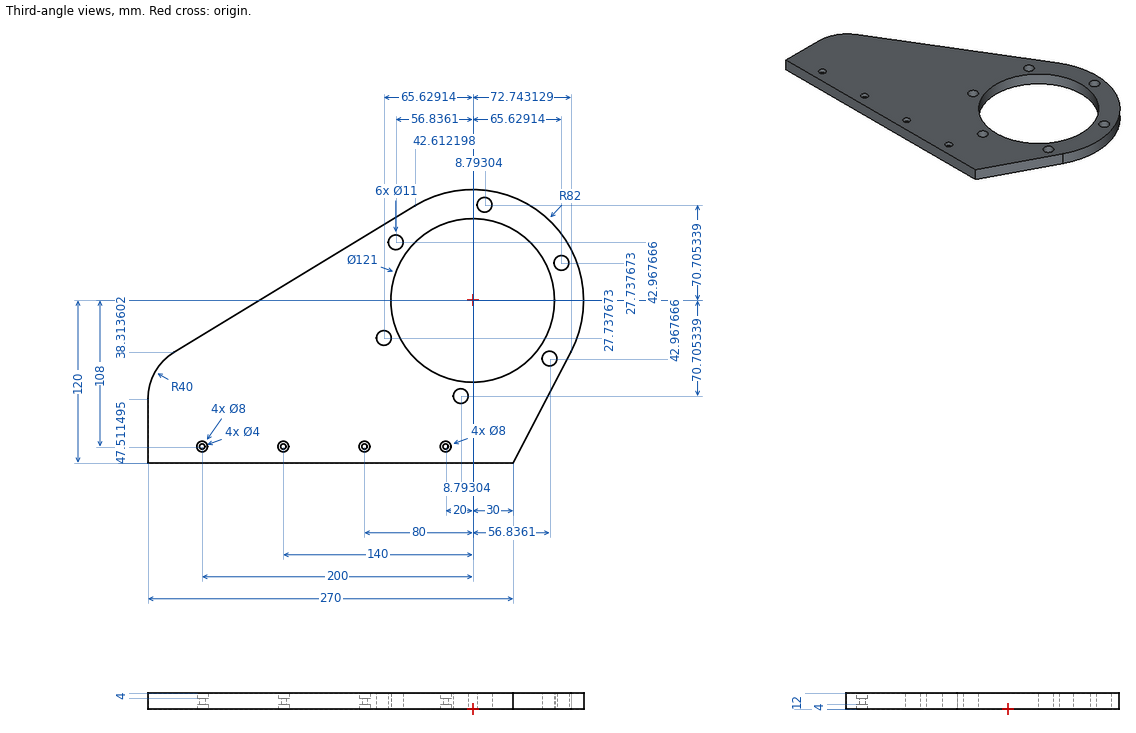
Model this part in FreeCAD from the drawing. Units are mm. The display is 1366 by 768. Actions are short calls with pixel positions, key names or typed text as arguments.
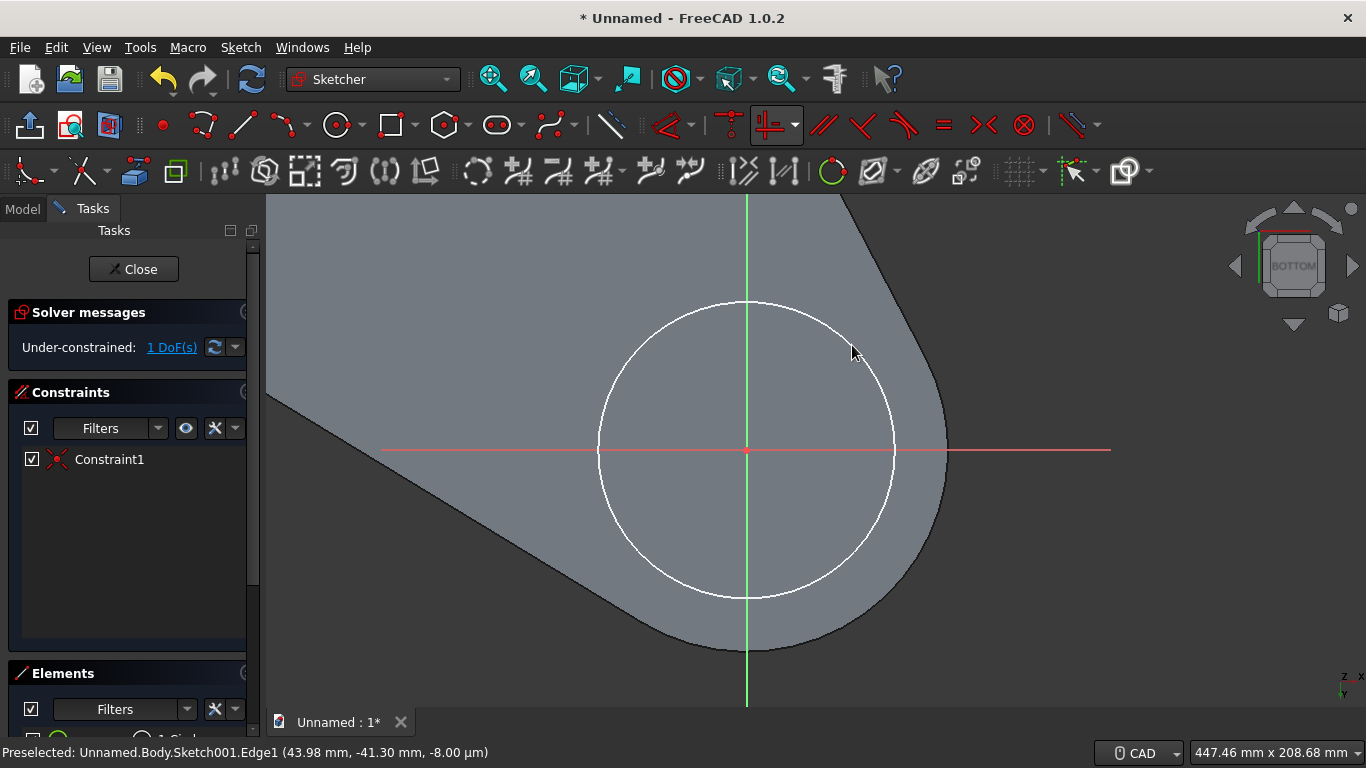
click(666, 126)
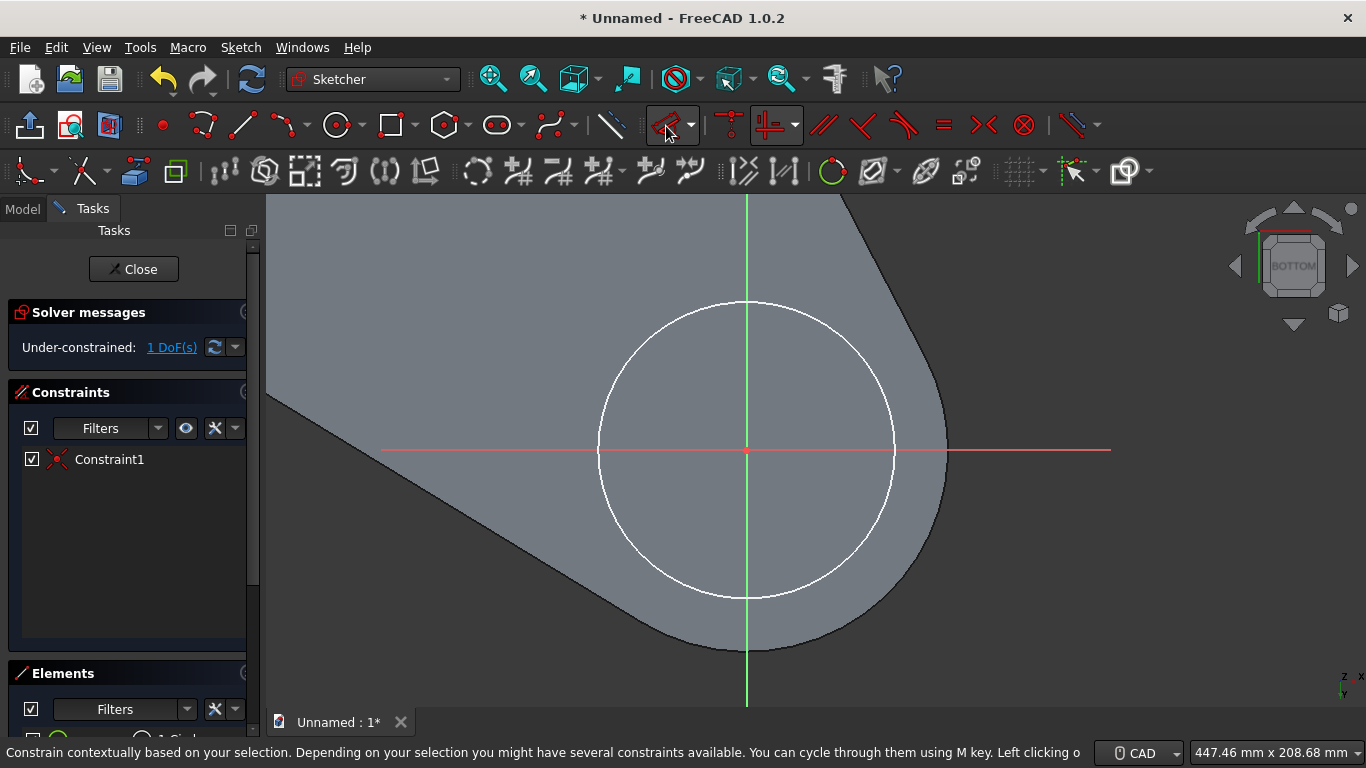
click(851, 345)
click(874, 322)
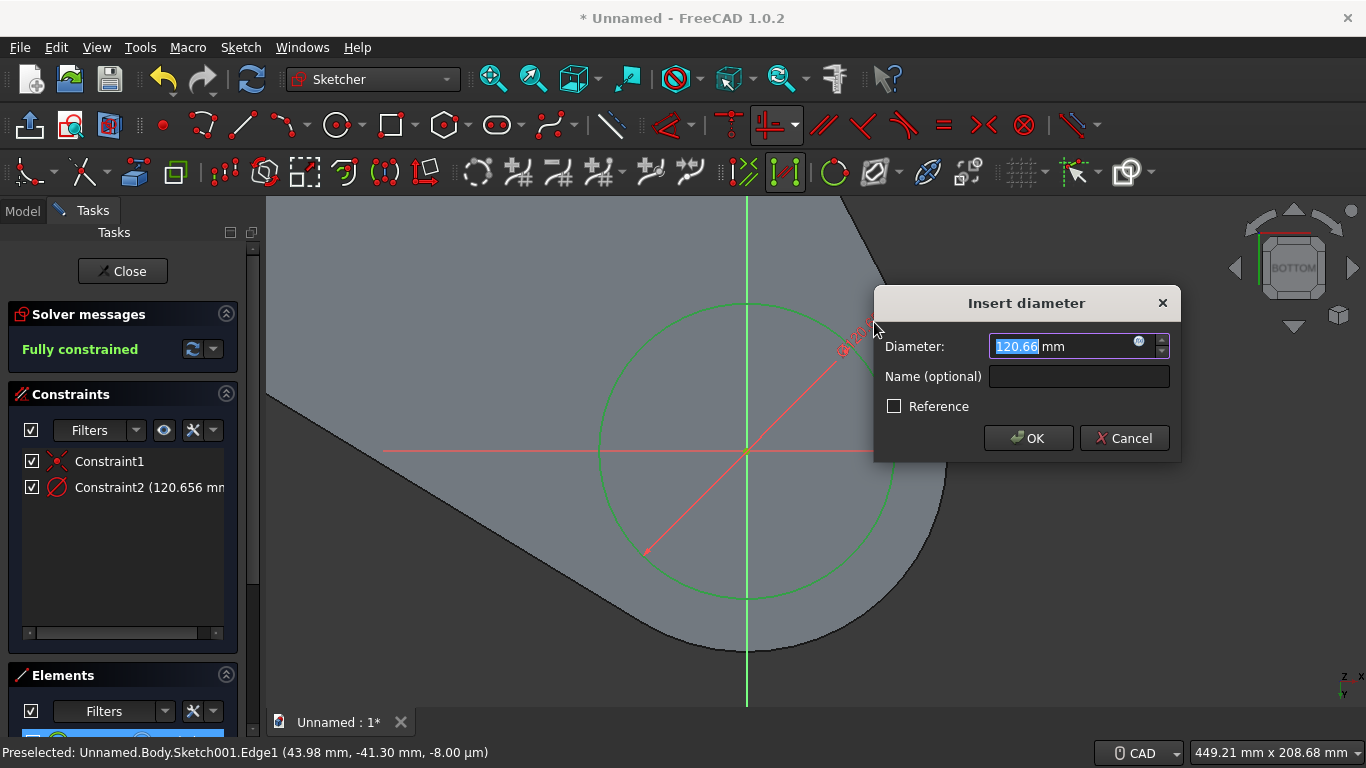
text(121)
key(Return)
key(Escape)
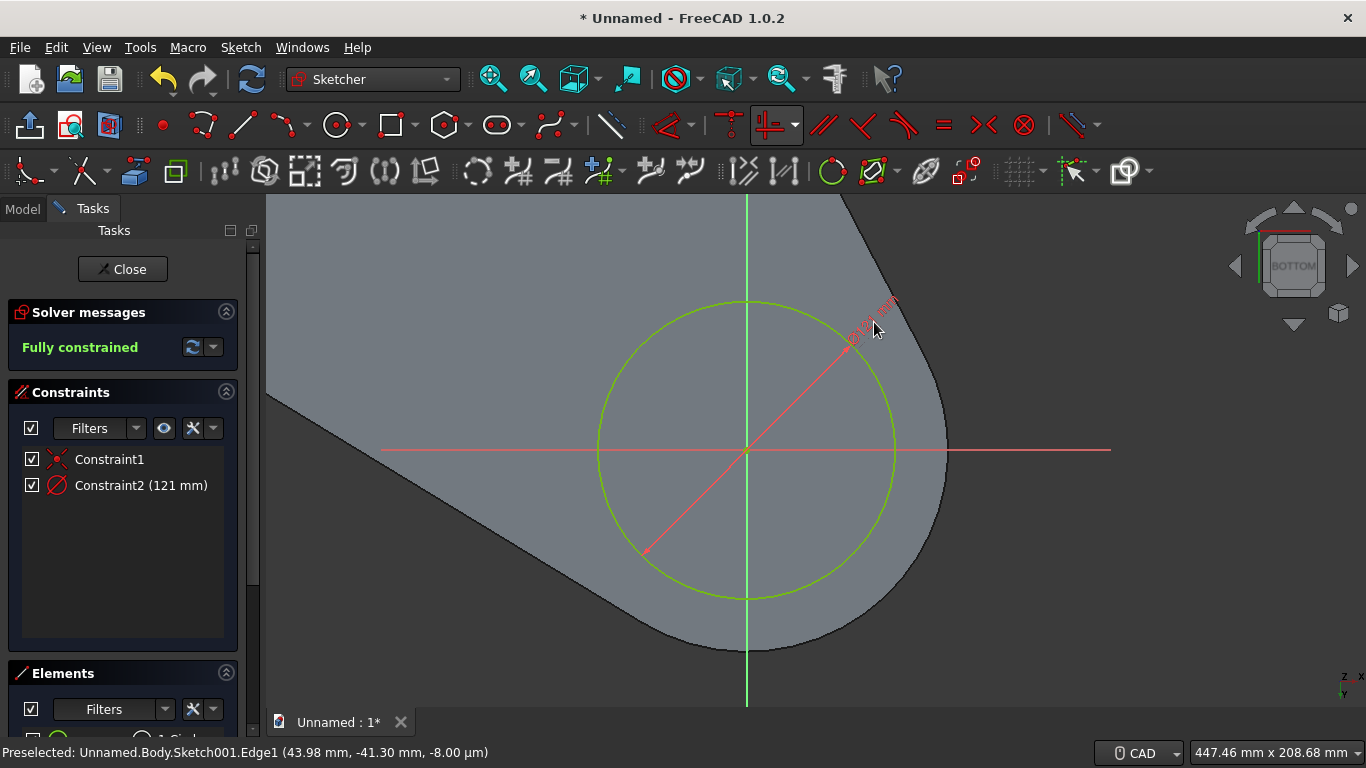
click(123, 269)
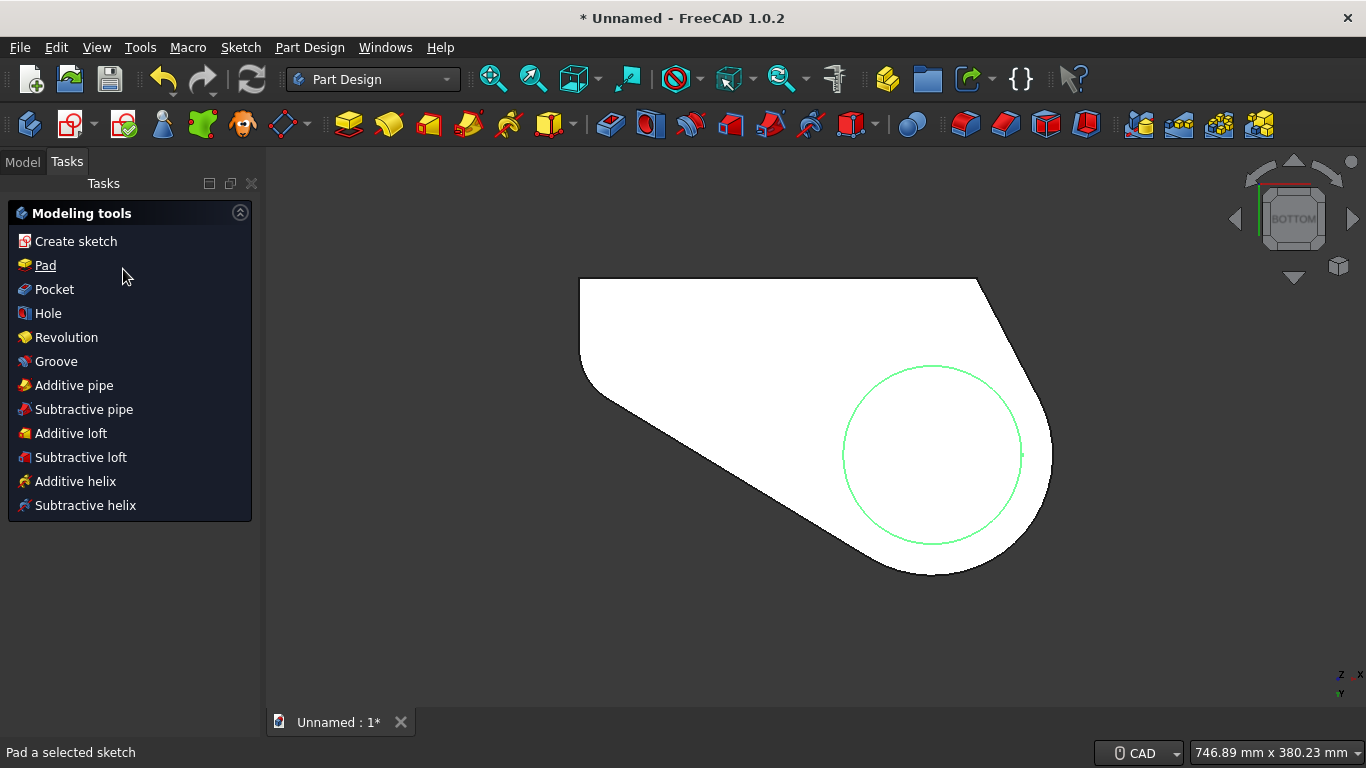
click(612, 124)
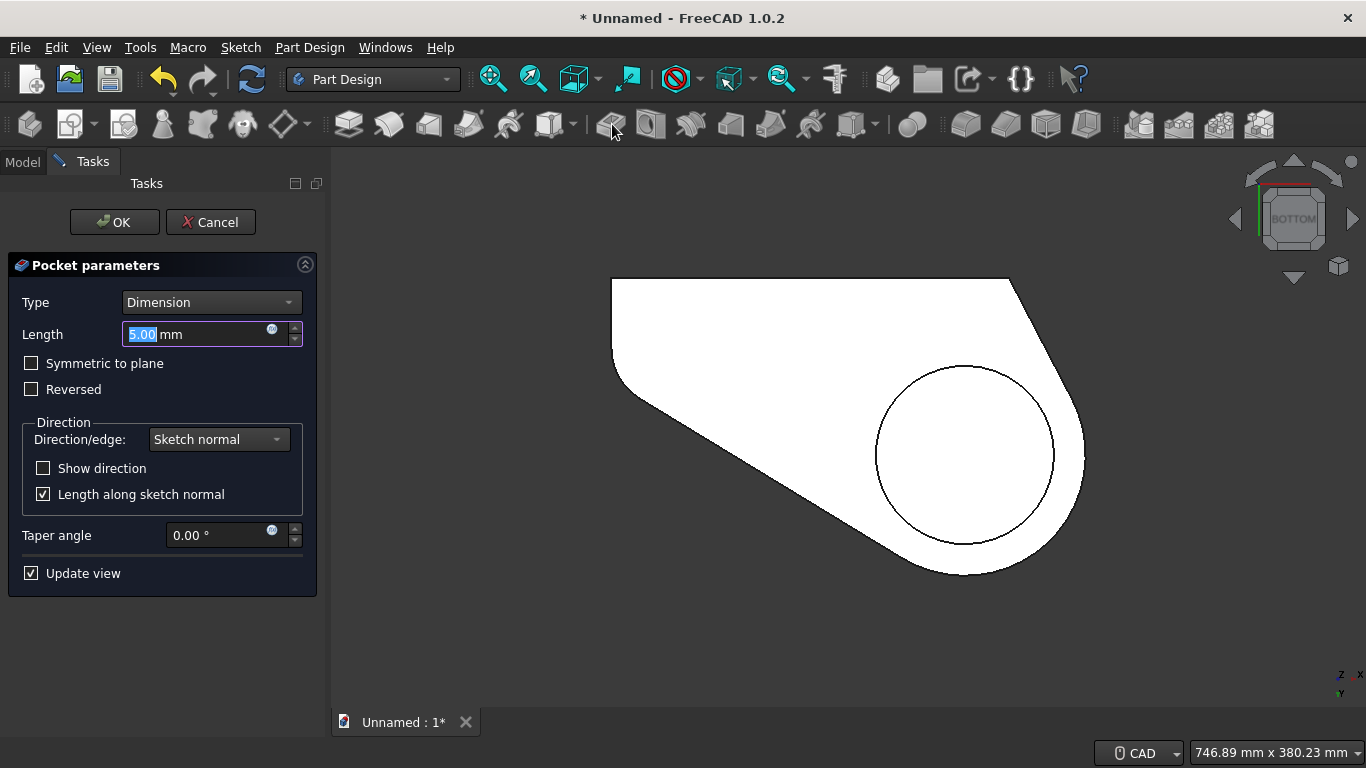
click(212, 302)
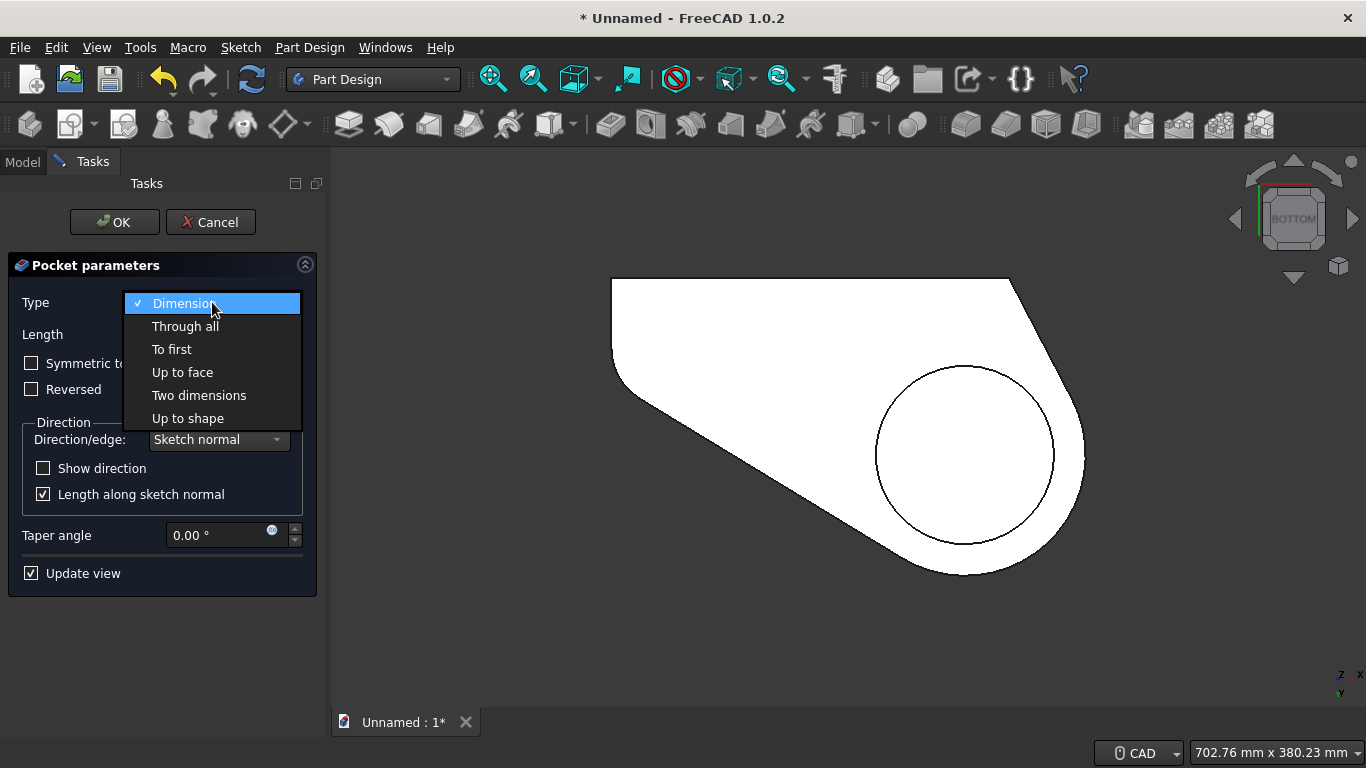
click(212, 326)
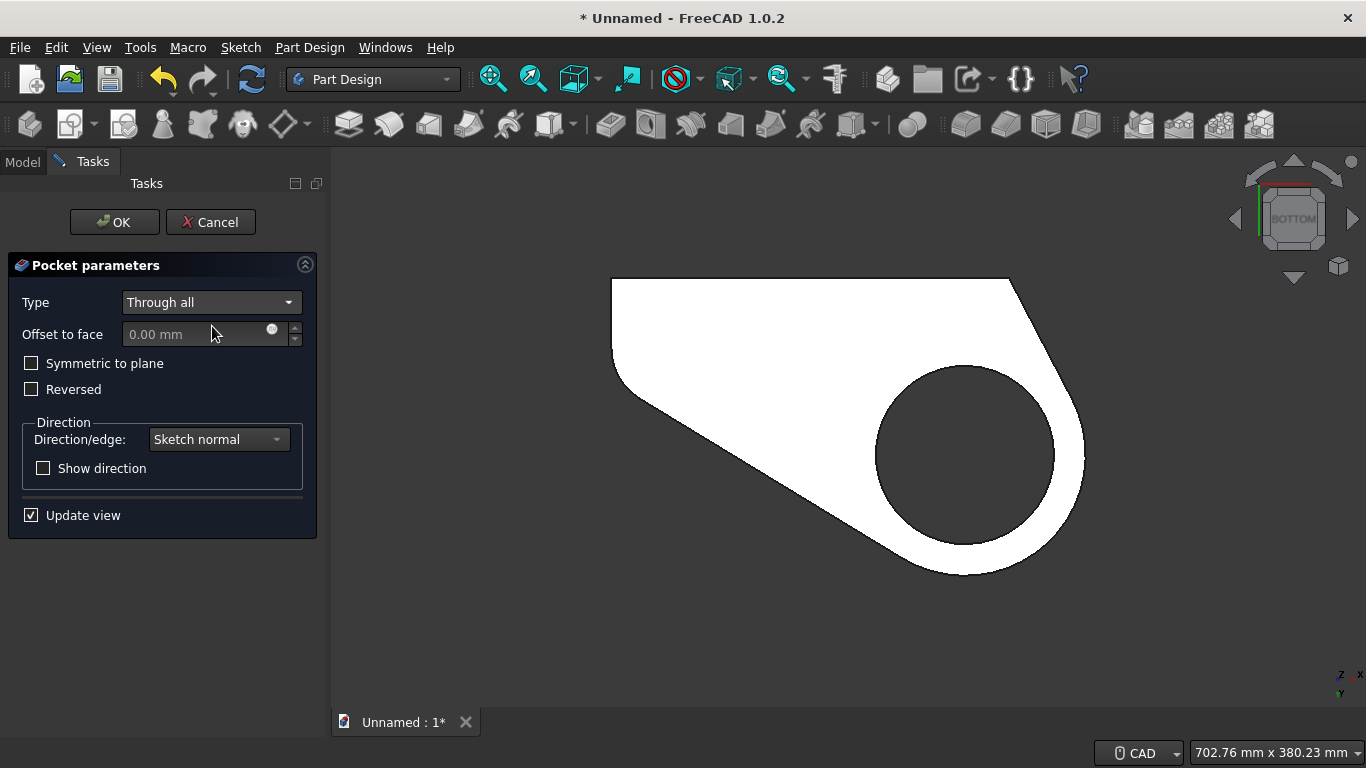
click(115, 222)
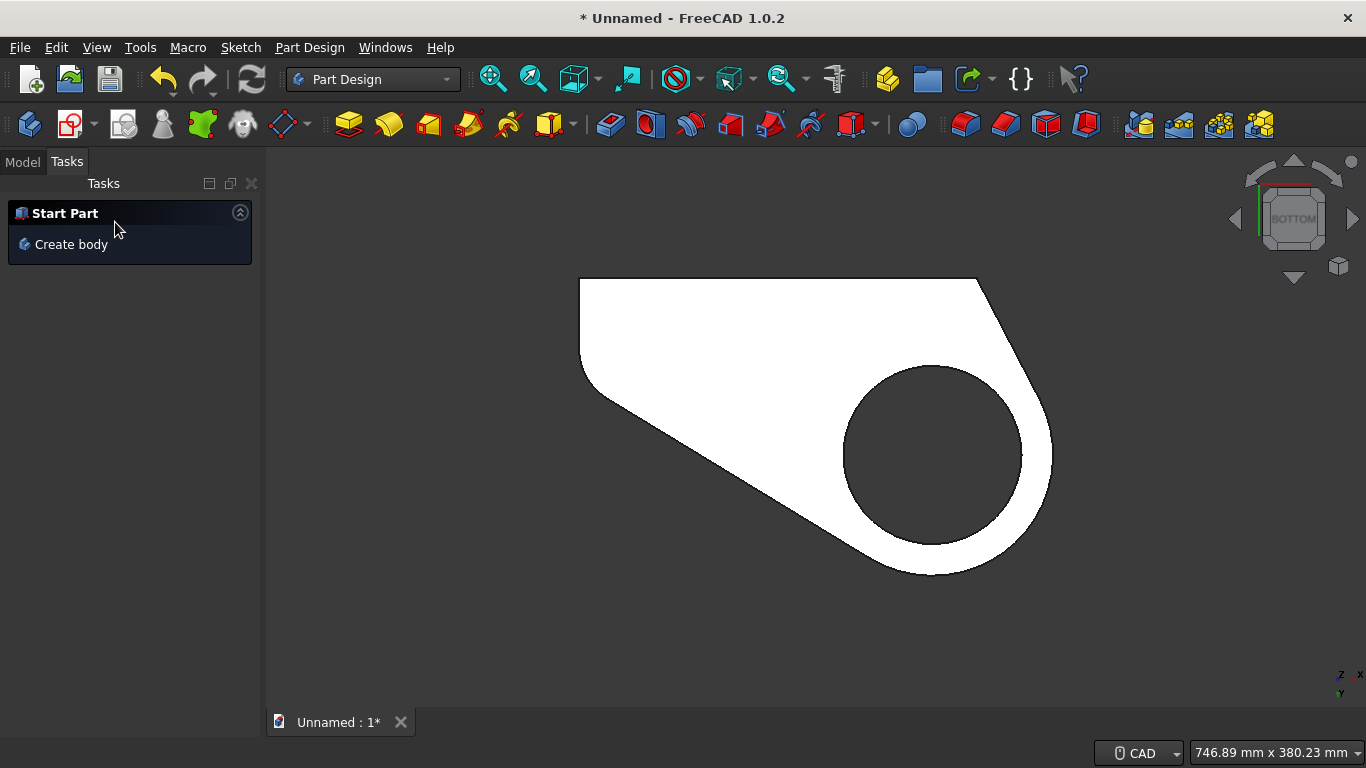
key(0)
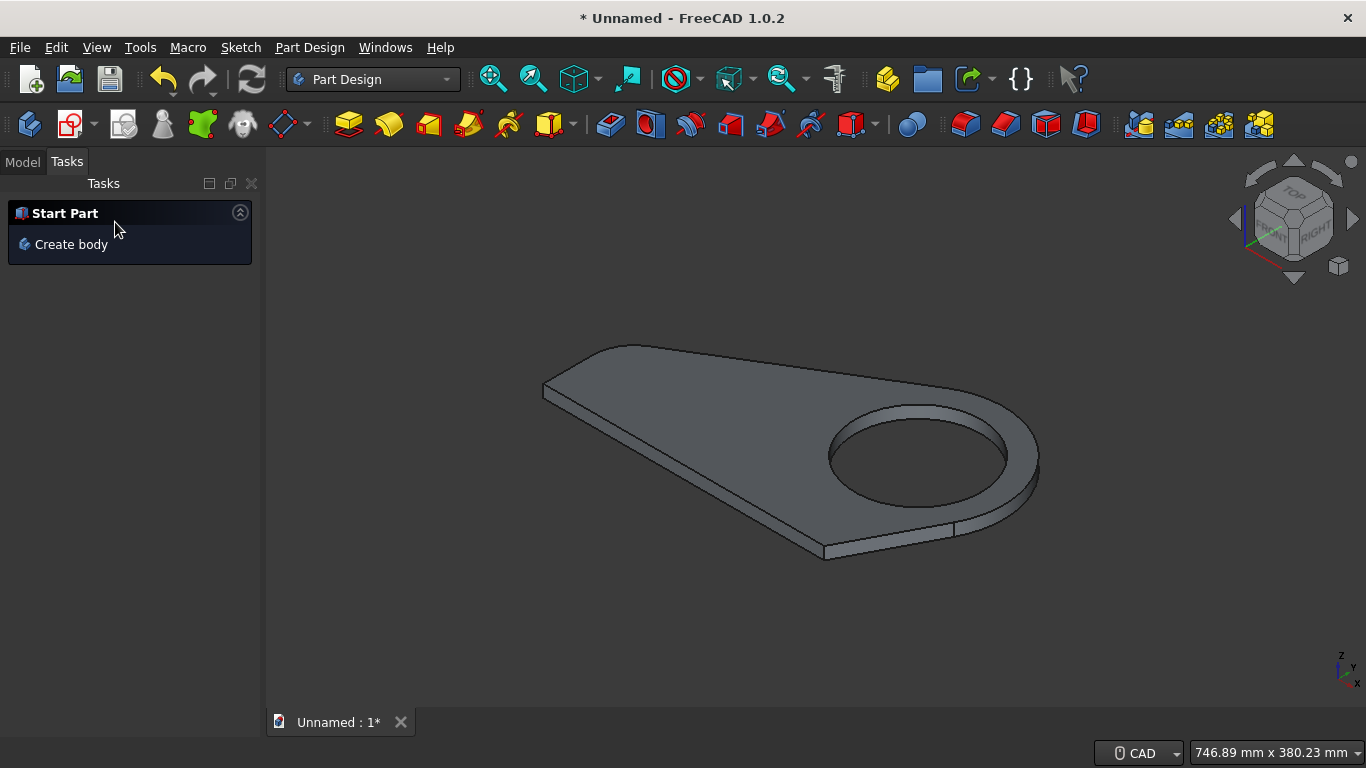
click(738, 408)